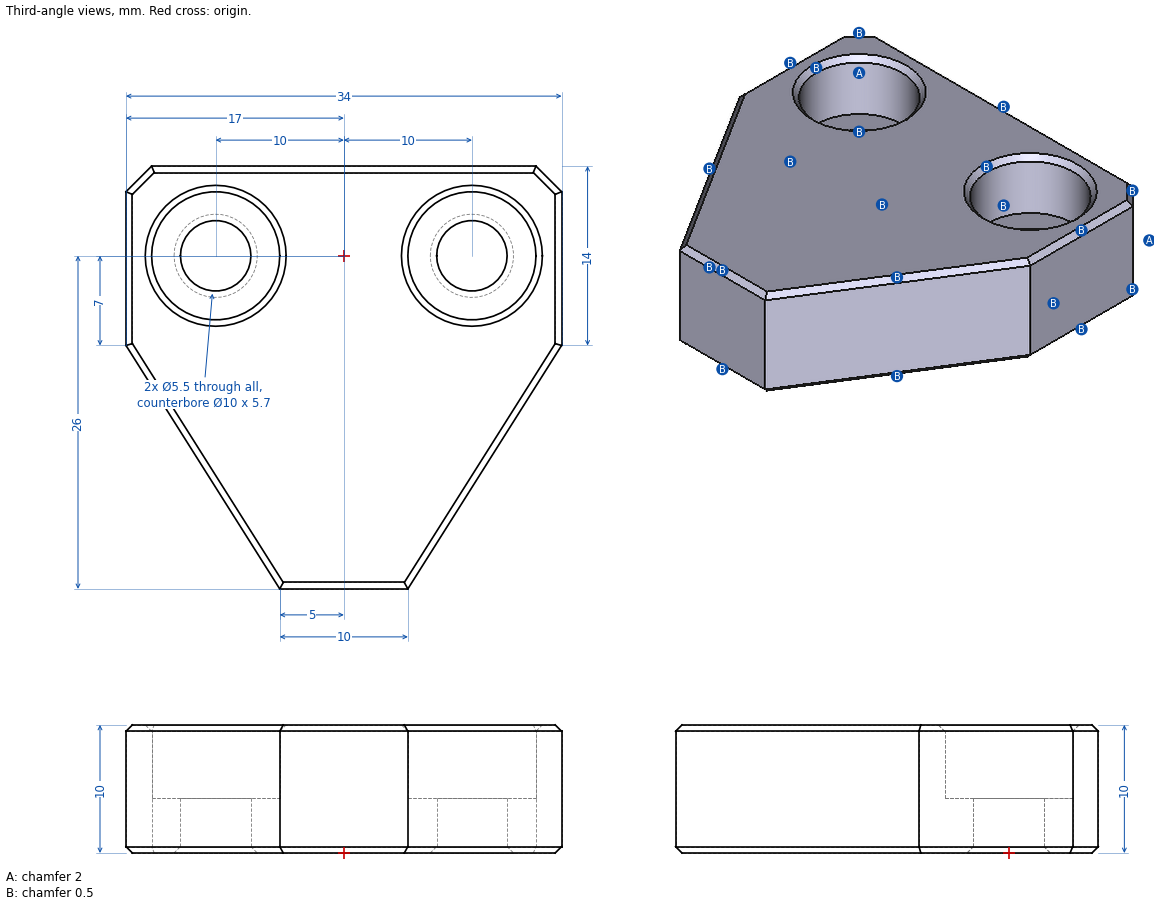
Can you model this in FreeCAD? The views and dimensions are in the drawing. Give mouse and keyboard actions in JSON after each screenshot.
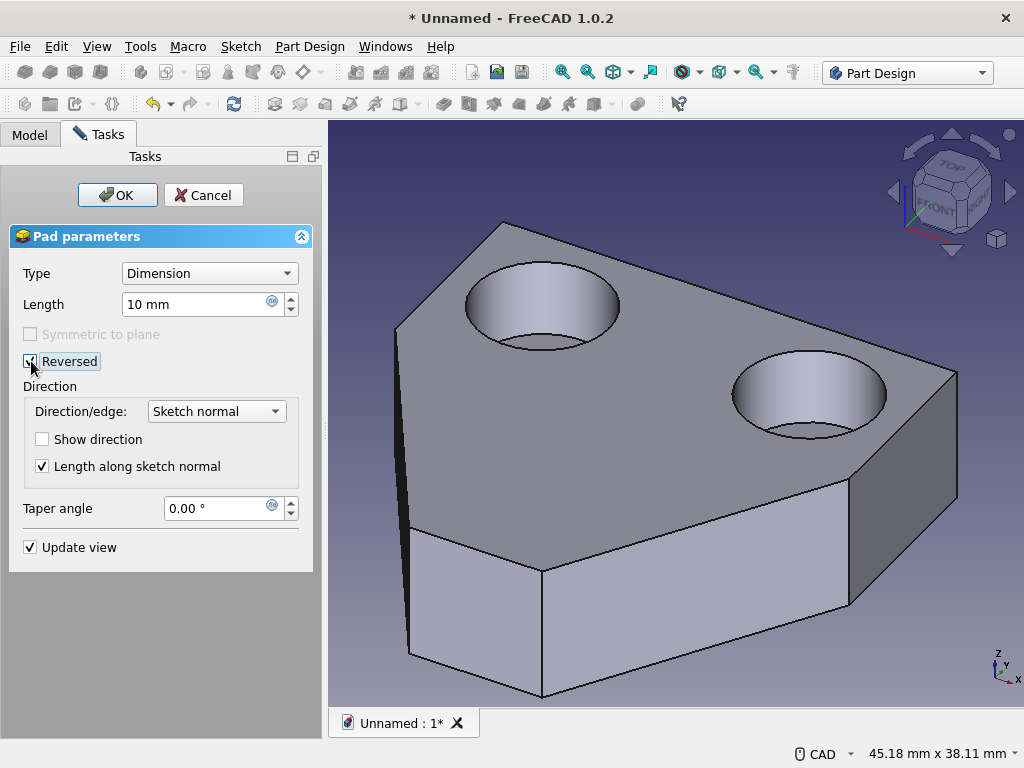
{"action": "left_click", "coordinate": [118, 195]}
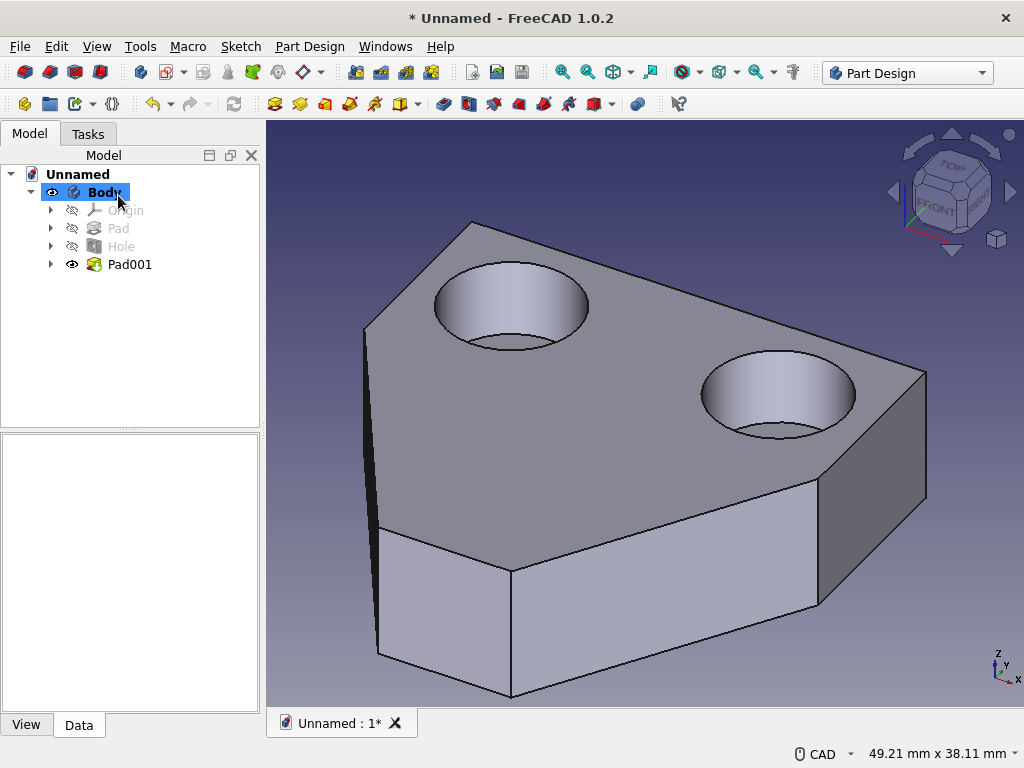
{"action": "left_click", "coordinate": [563, 72]}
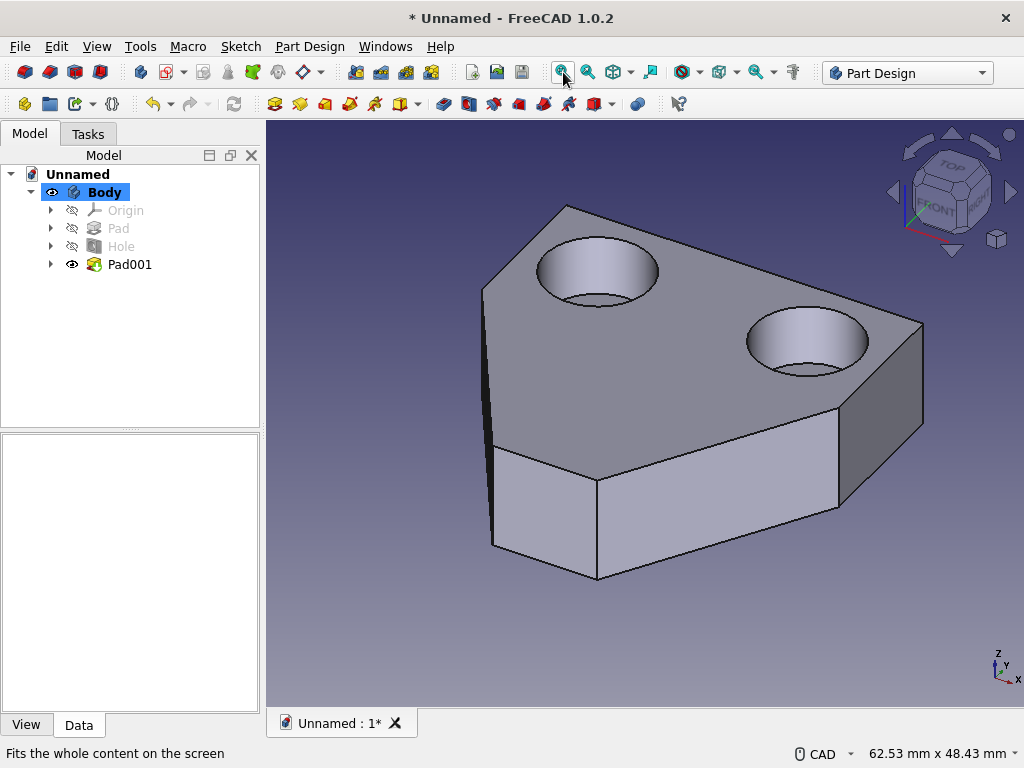
{"action": "key", "text": "0"}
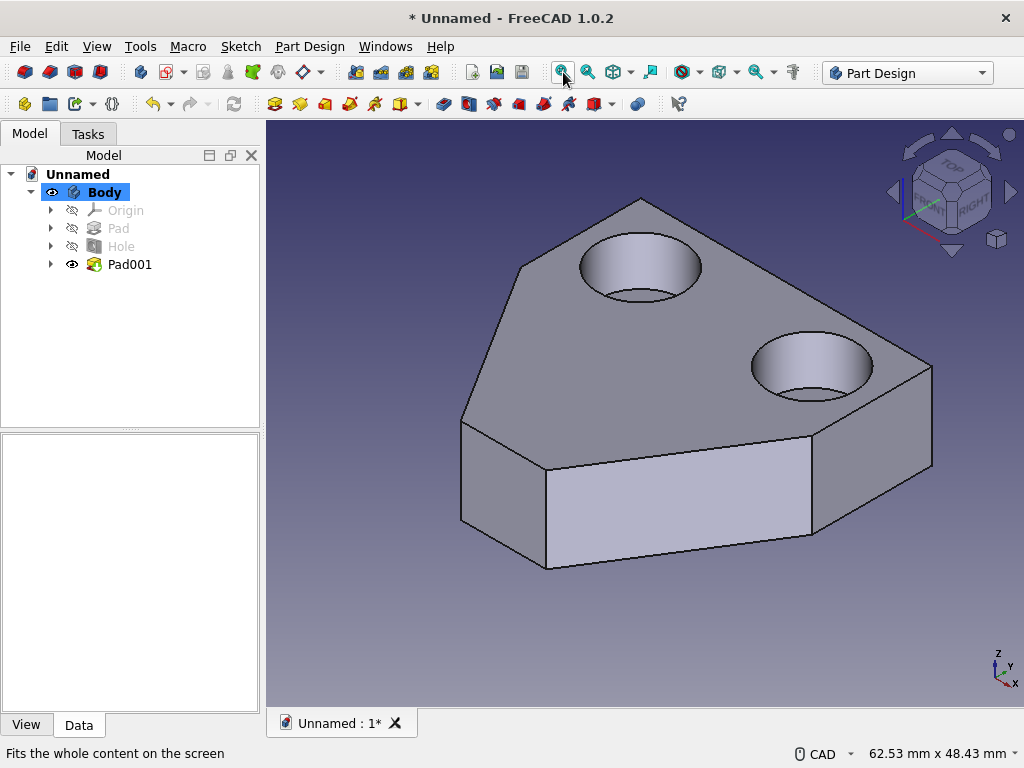
{"action": "key", "text": "2"}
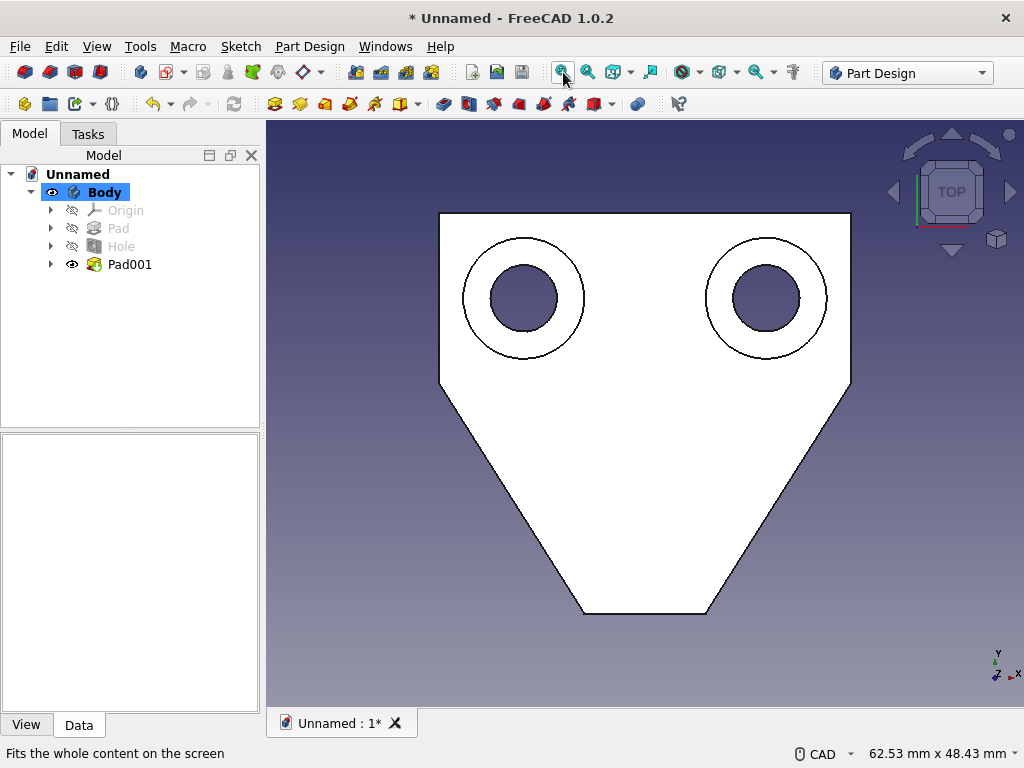
{"action": "key", "text": "1"}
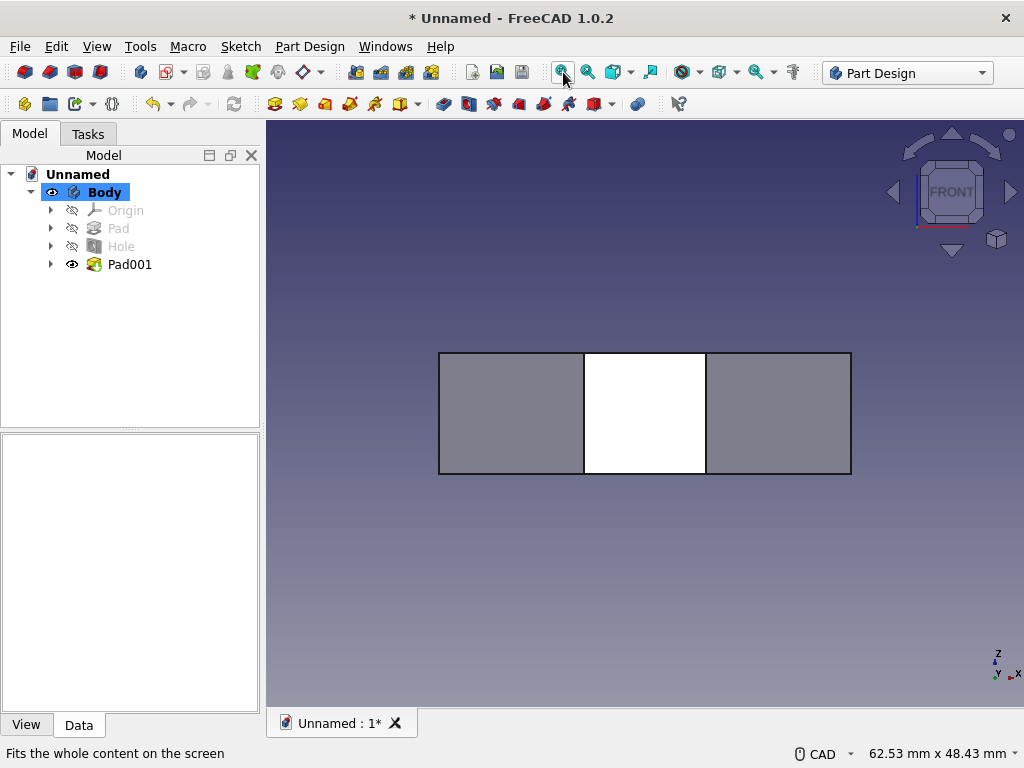
{"action": "key", "text": "3"}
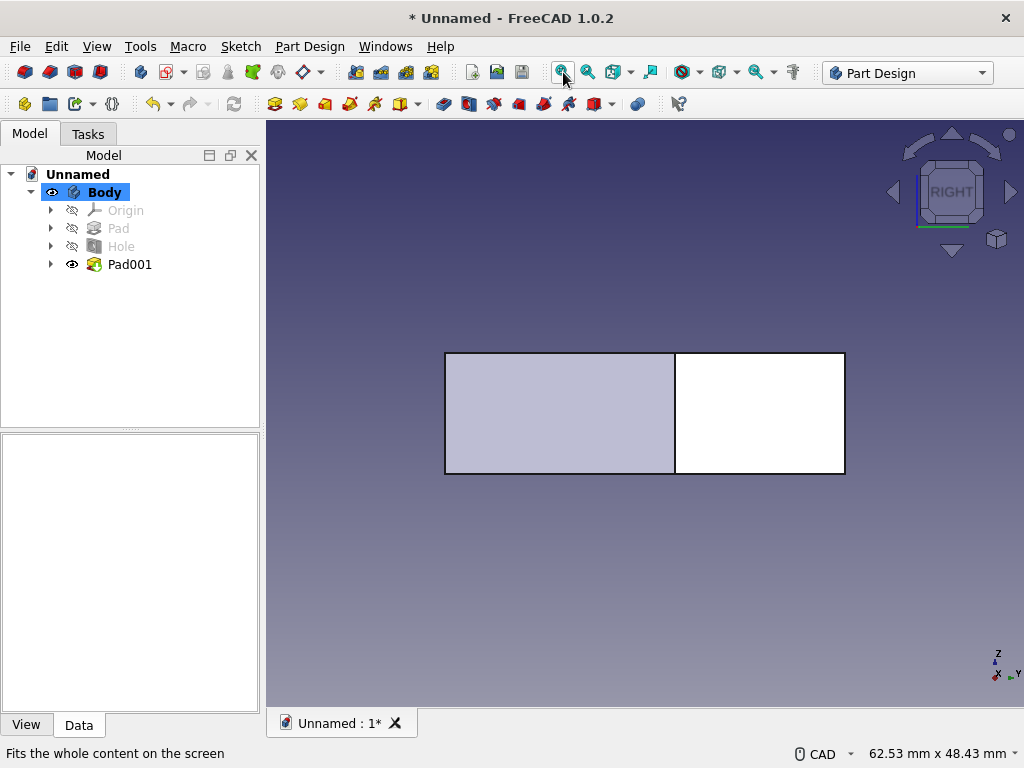
{"action": "left_click", "coordinate": [845, 412]}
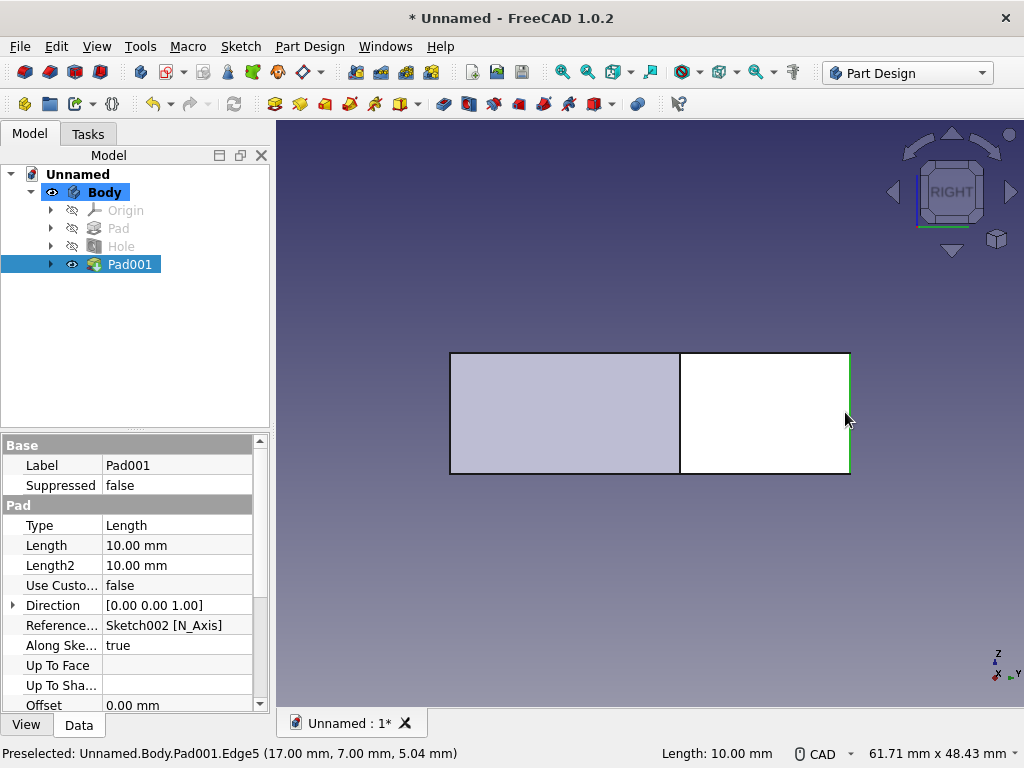
{"action": "key", "text": "5"}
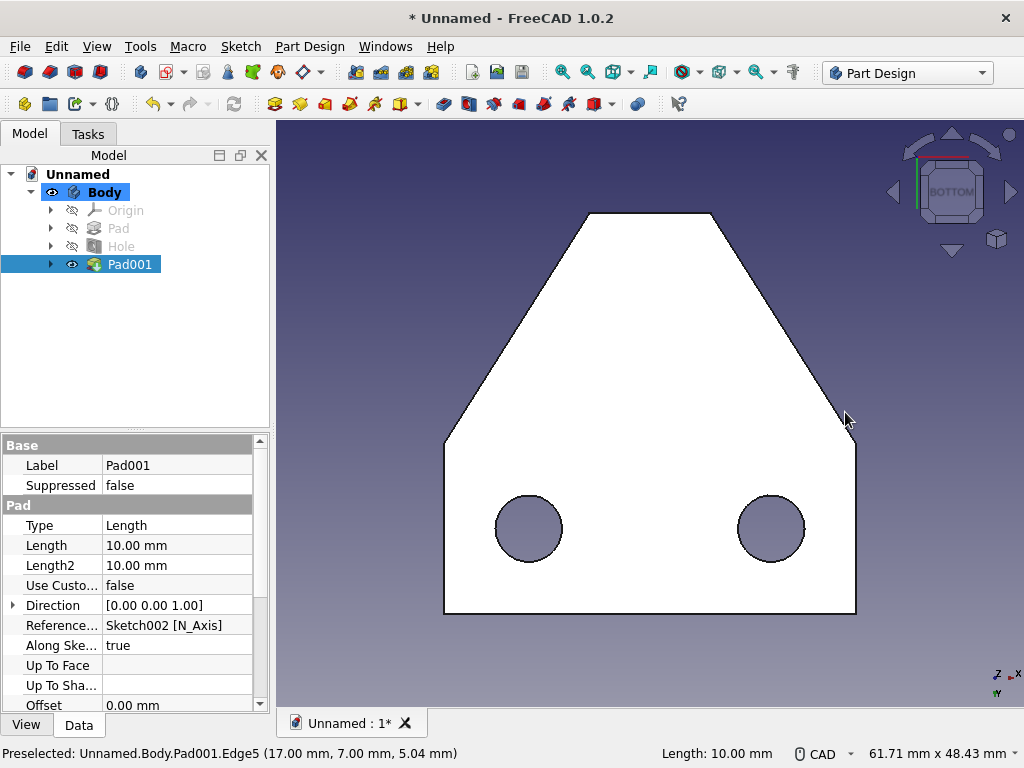
{"action": "key", "text": "4"}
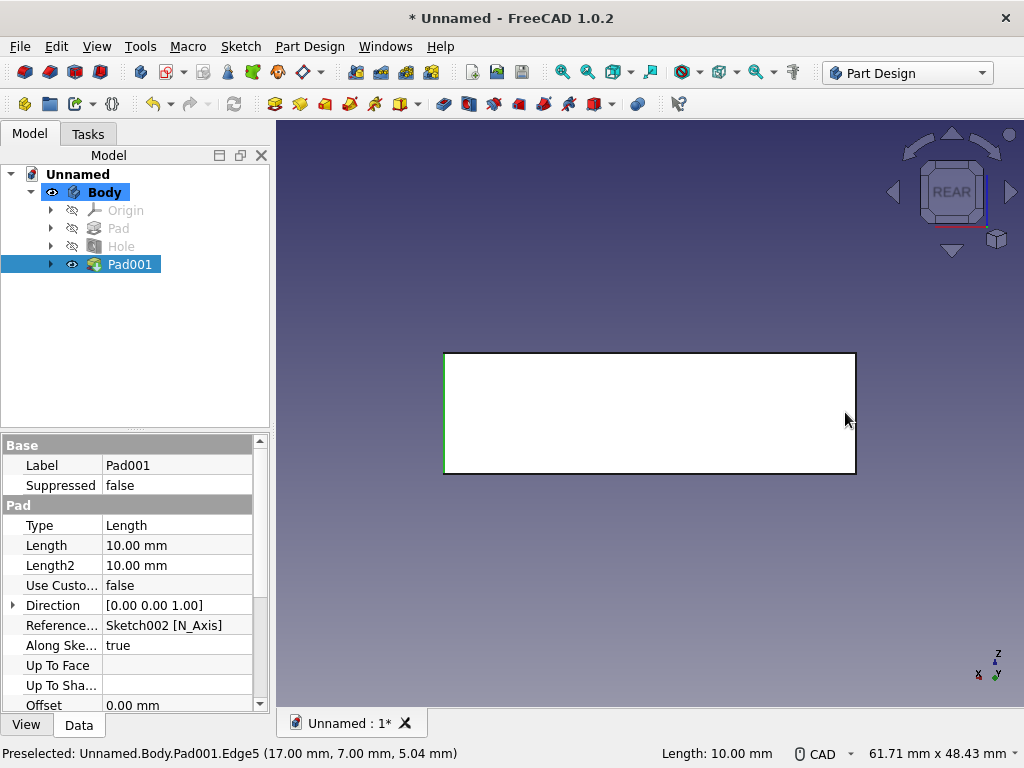
{"action": "left_click", "coordinate": [856, 413], "text": "ctrl"}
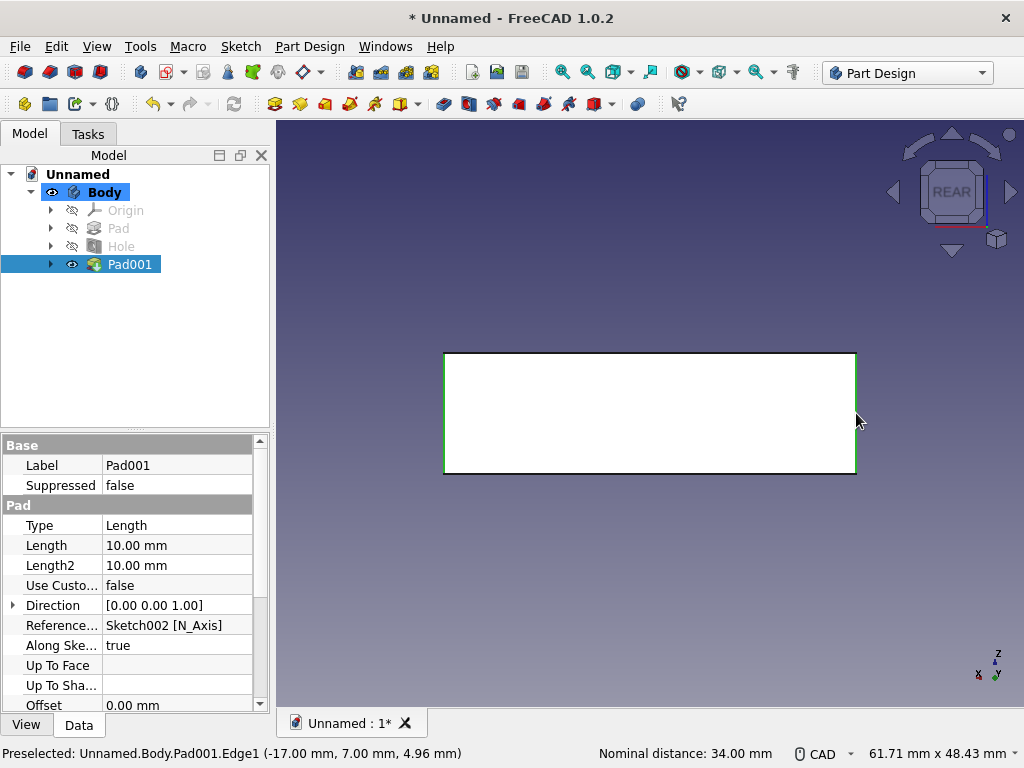
{"action": "left_click", "coordinate": [50, 72]}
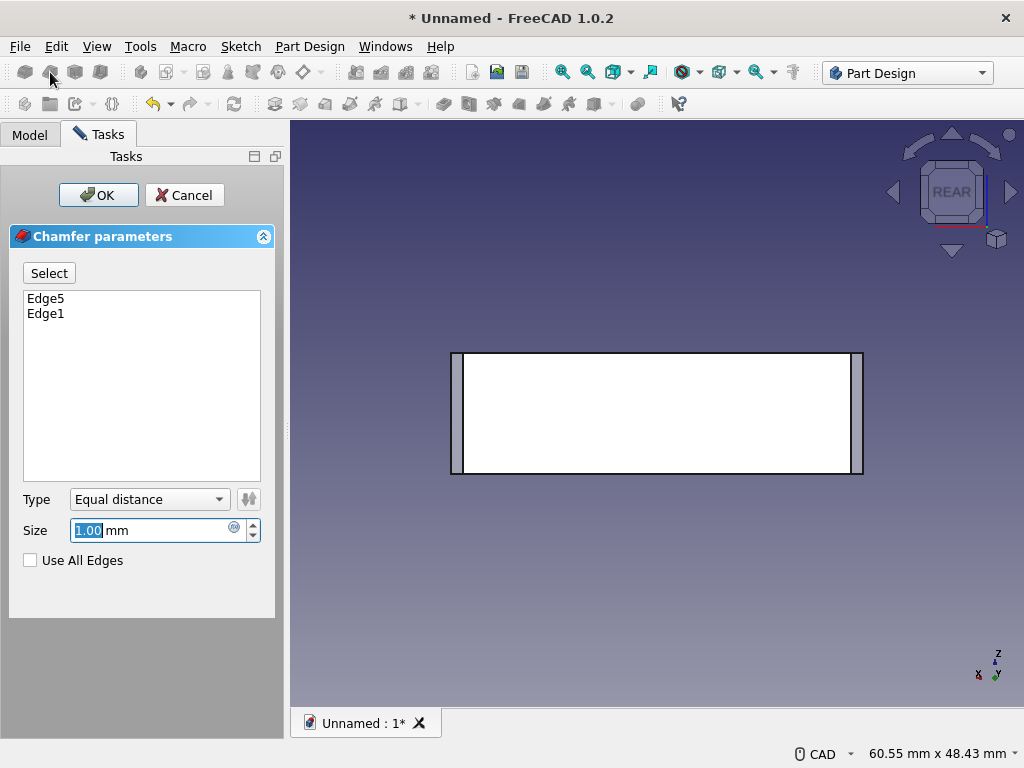
{"action": "type", "text": "2"}
{"action": "key", "text": "Tab"}